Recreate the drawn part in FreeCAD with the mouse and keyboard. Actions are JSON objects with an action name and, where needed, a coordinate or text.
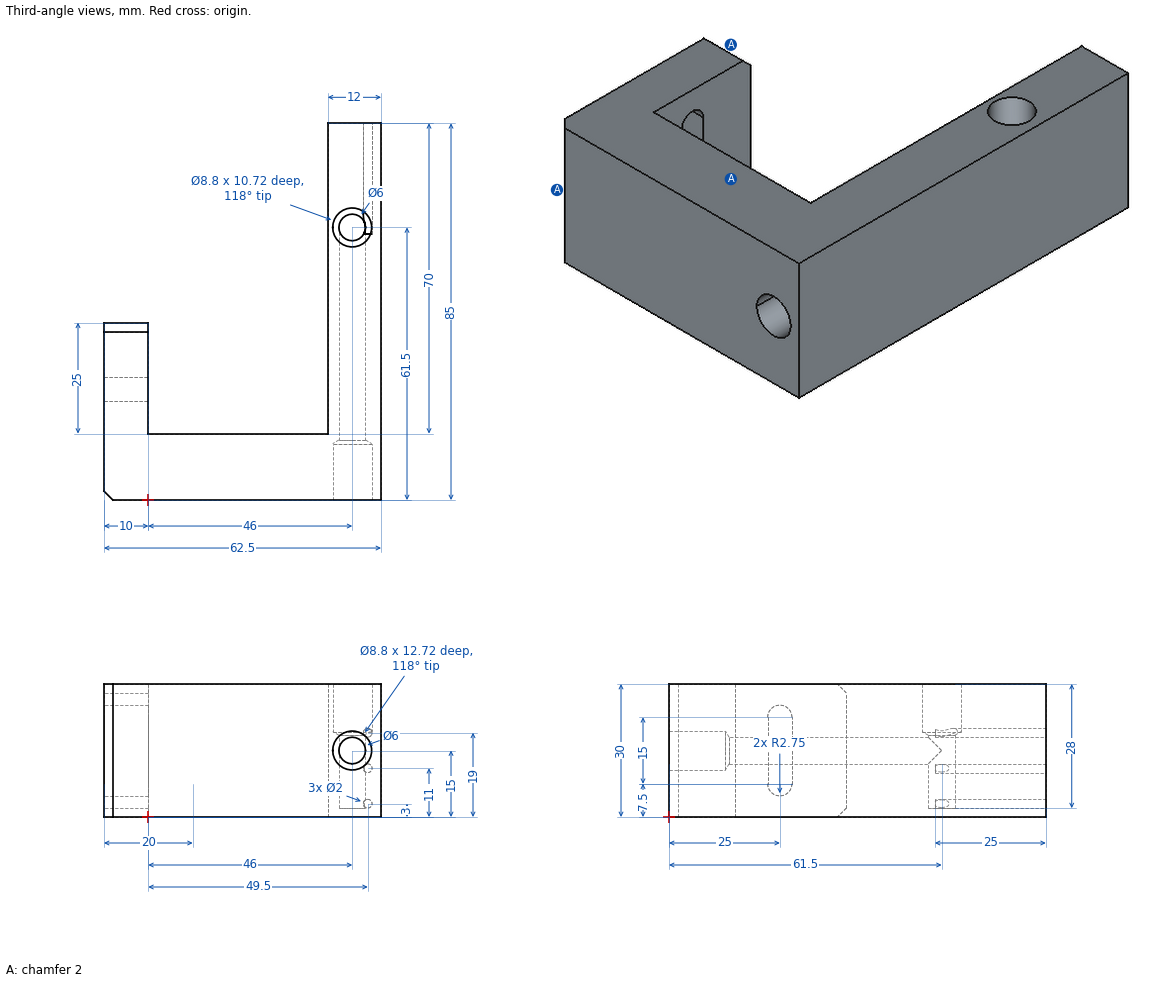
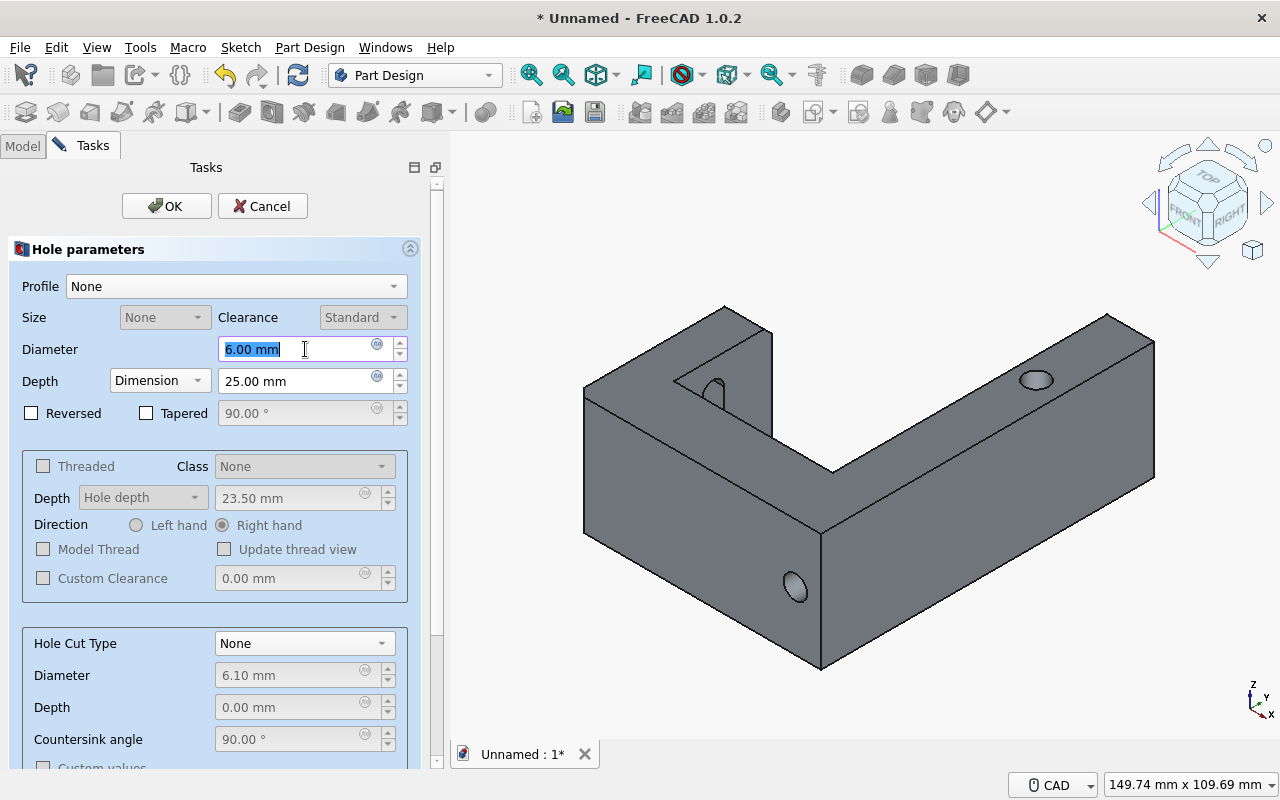
{"action": "type", "text": "8.8"}
{"action": "key", "text": "Tab"}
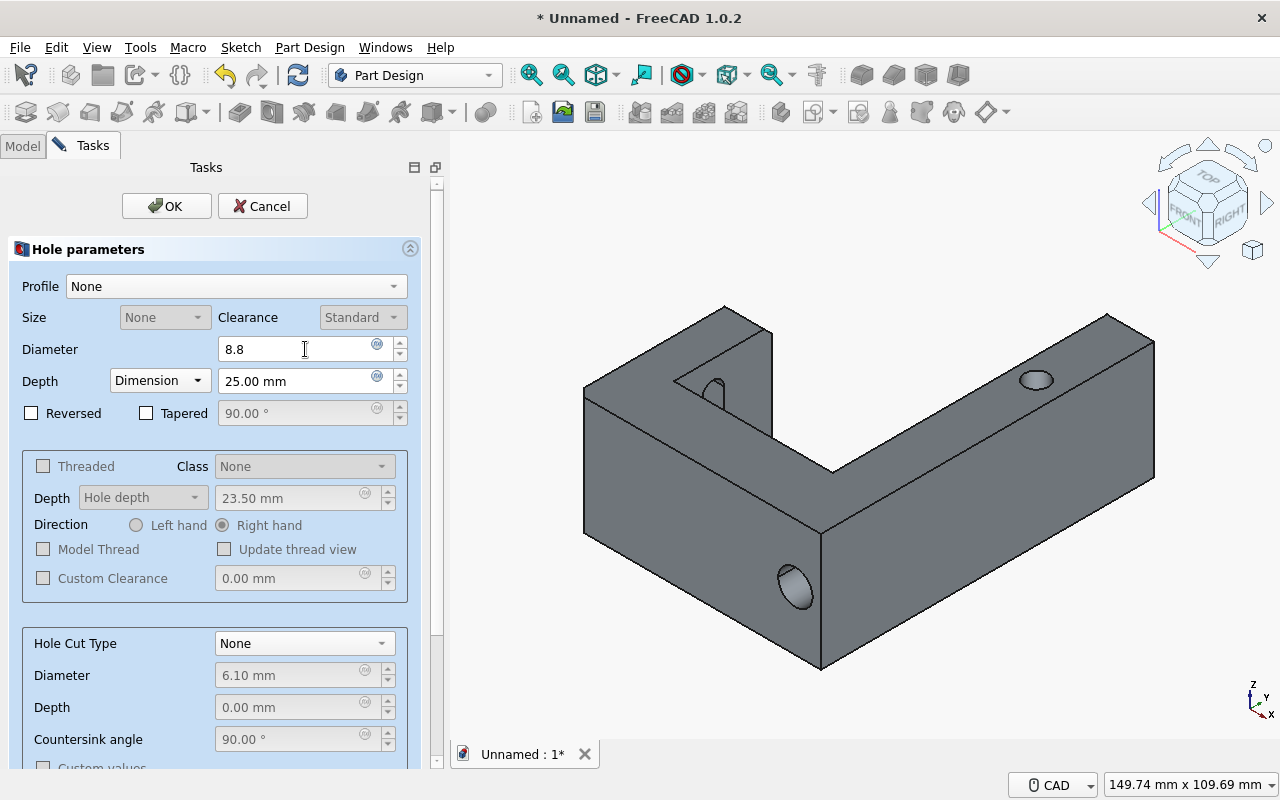
{"action": "triple_click", "coordinate": [305, 381]}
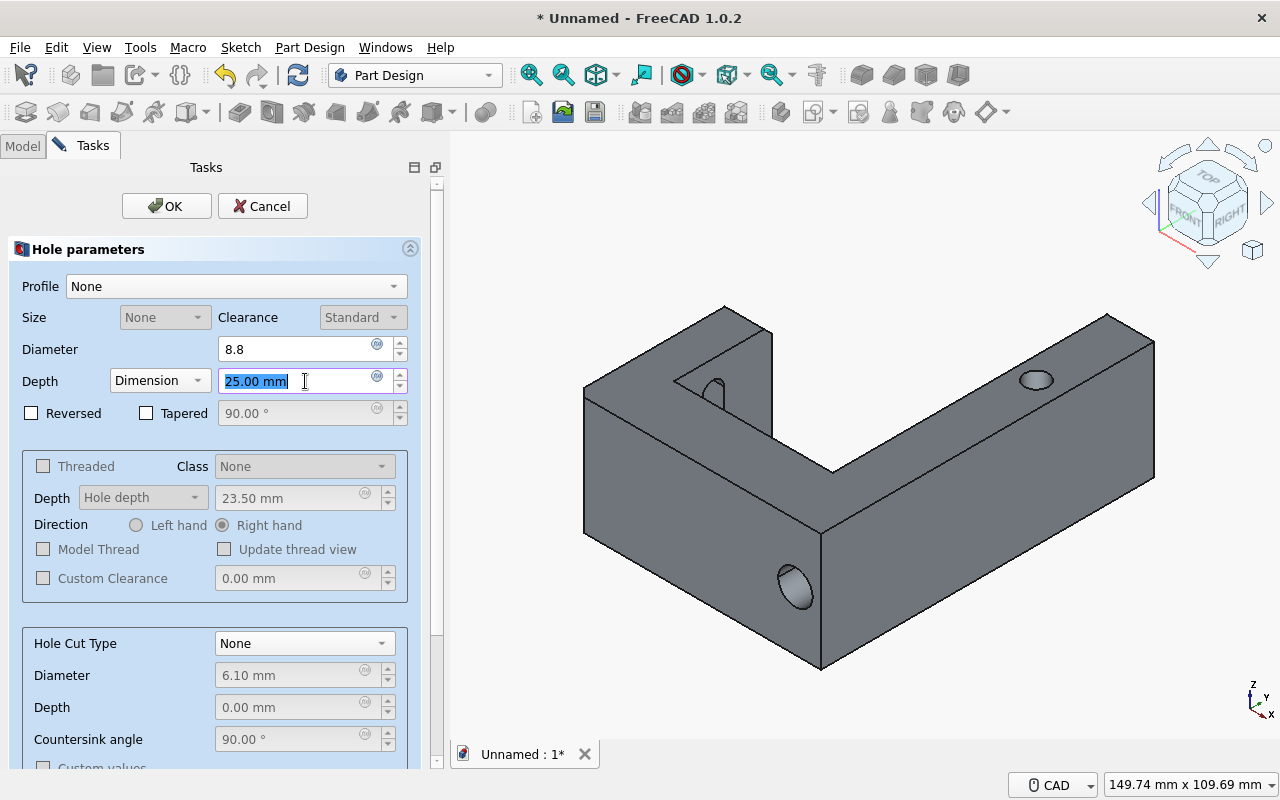
{"action": "type", "text": "12.72"}
{"action": "key", "text": "Tab"}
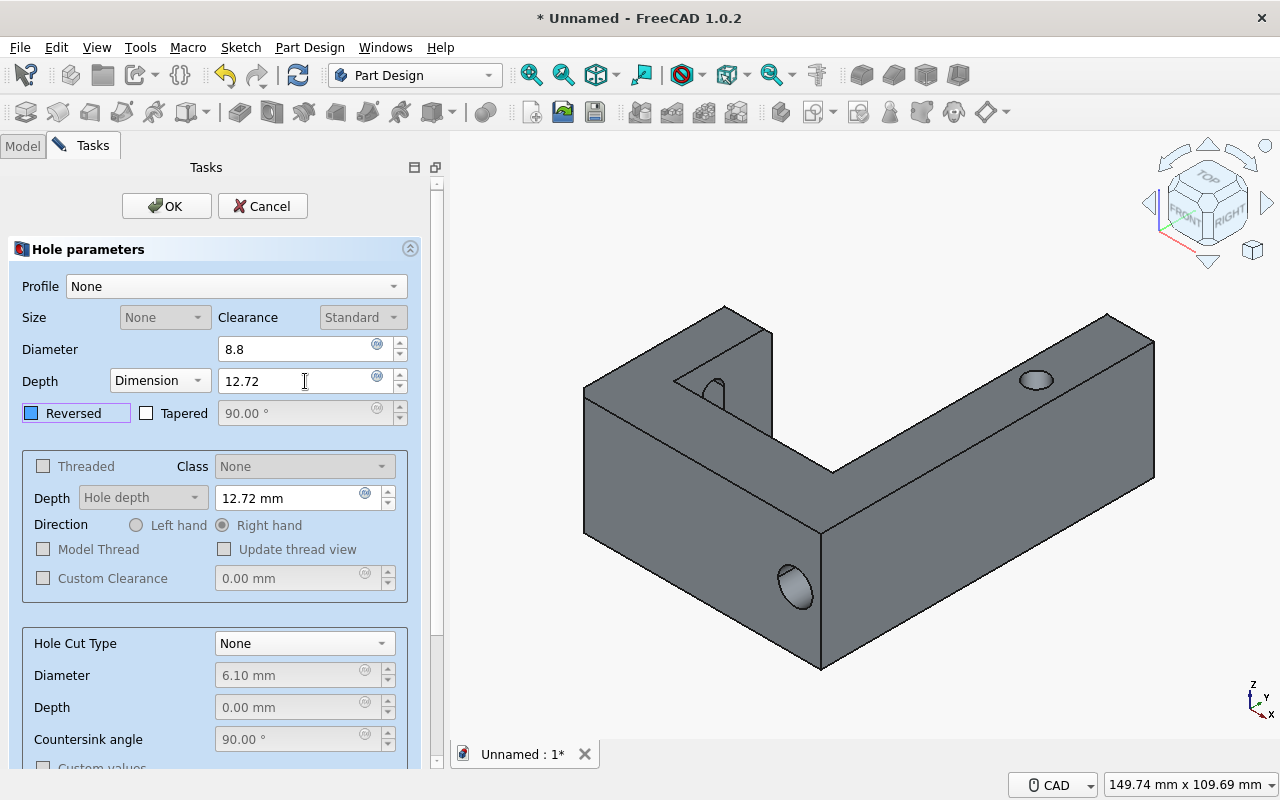
{"action": "left_click", "coordinate": [167, 206]}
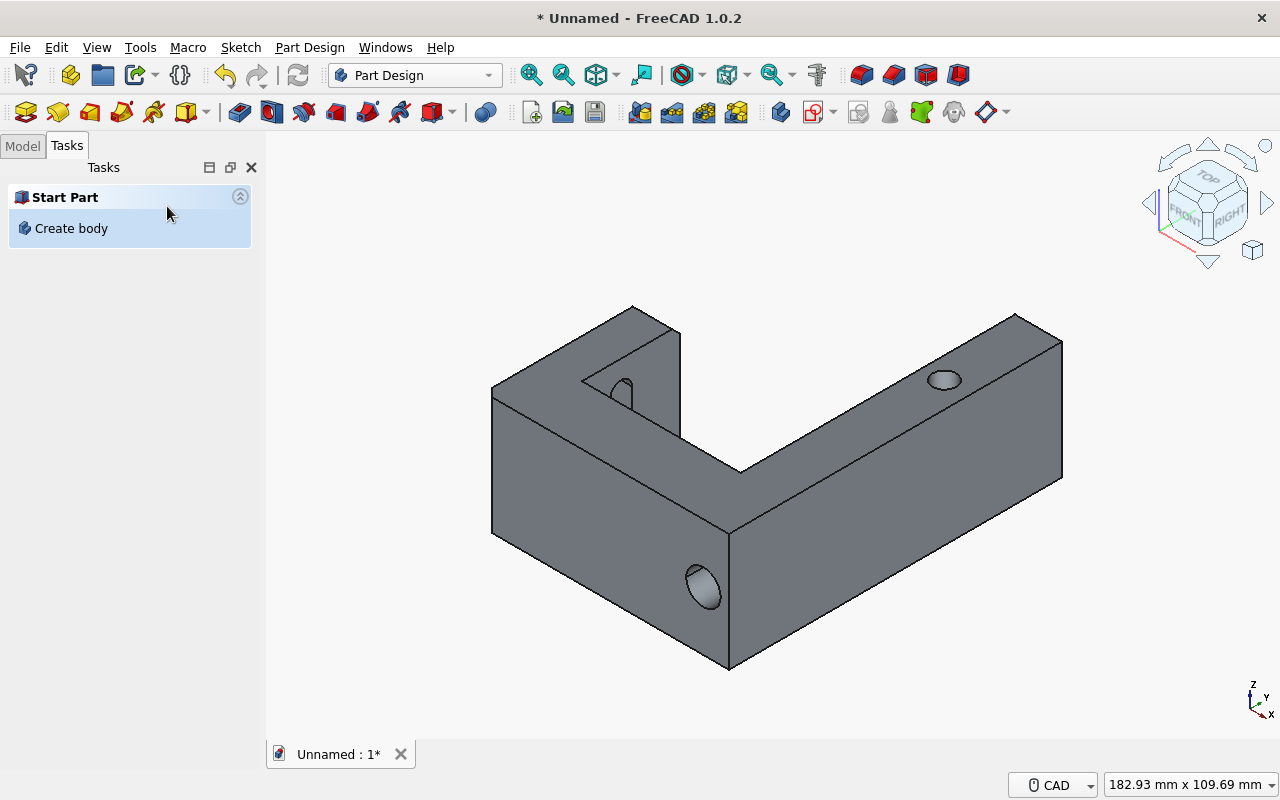
{"action": "left_click", "coordinate": [700, 489]}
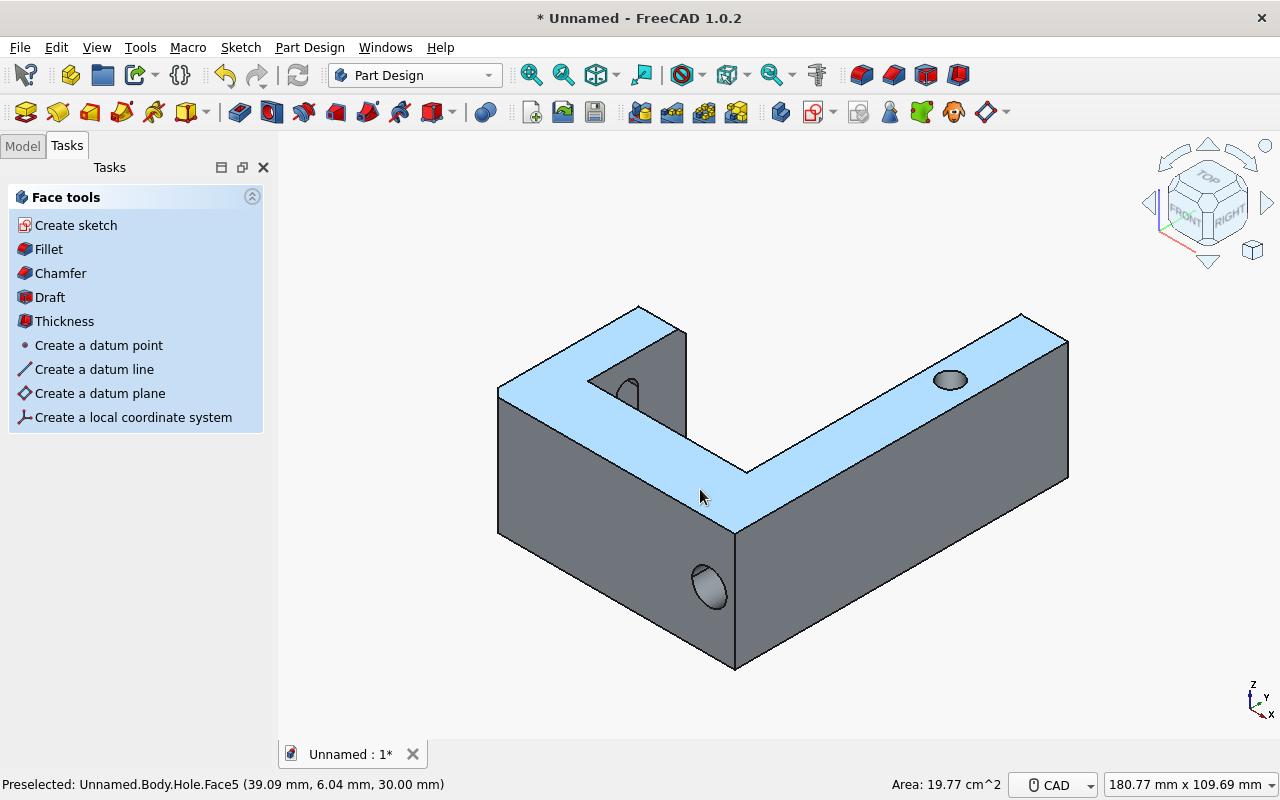
{"action": "left_click", "coordinate": [814, 112]}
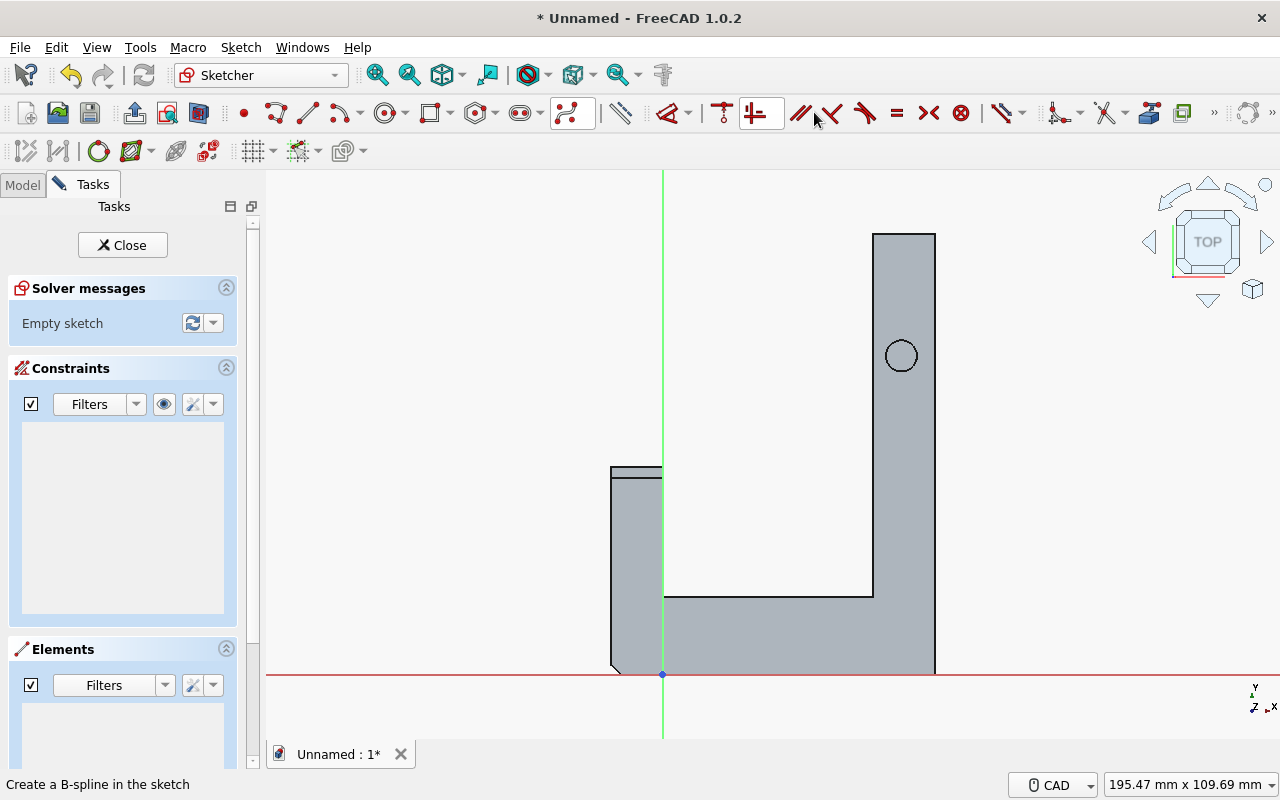
{"action": "scroll", "coordinate": [932, 341], "scroll_direction": "up", "scroll_amount": 10}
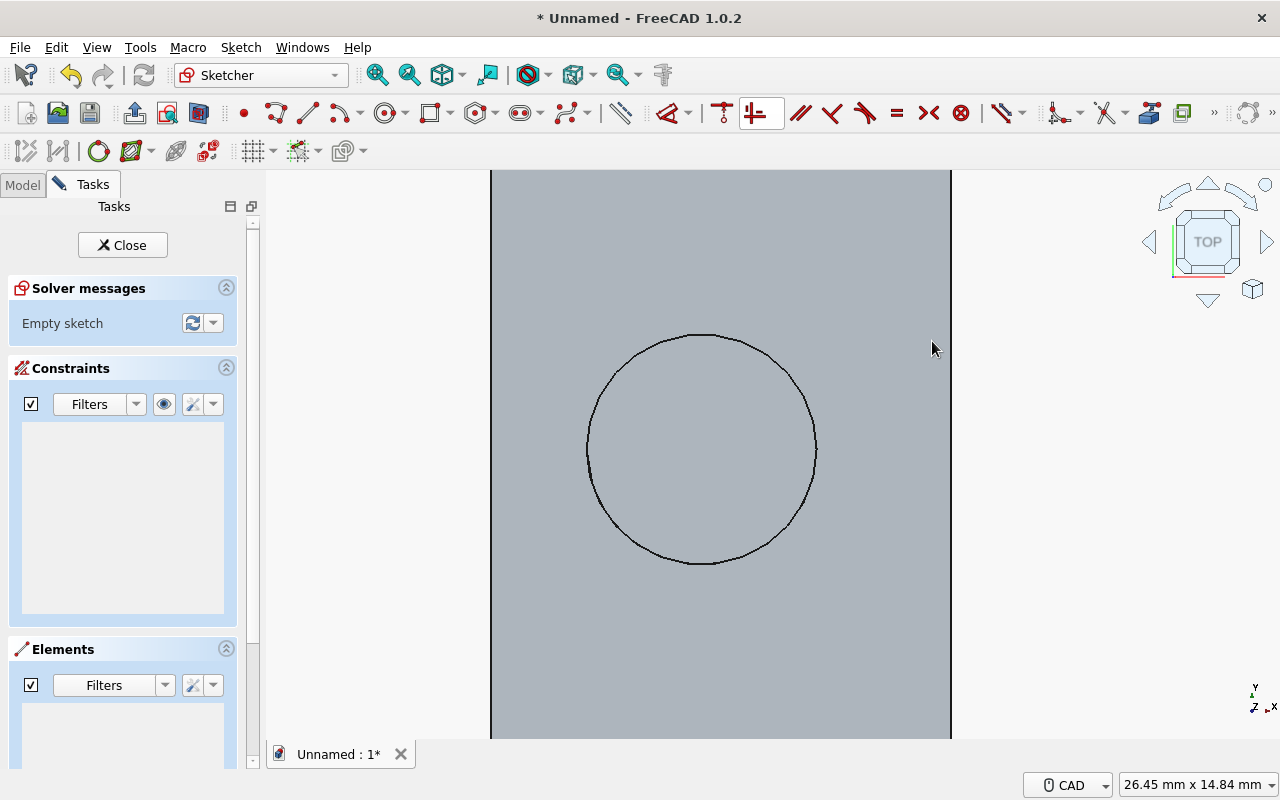
{"action": "left_click", "coordinate": [386, 114]}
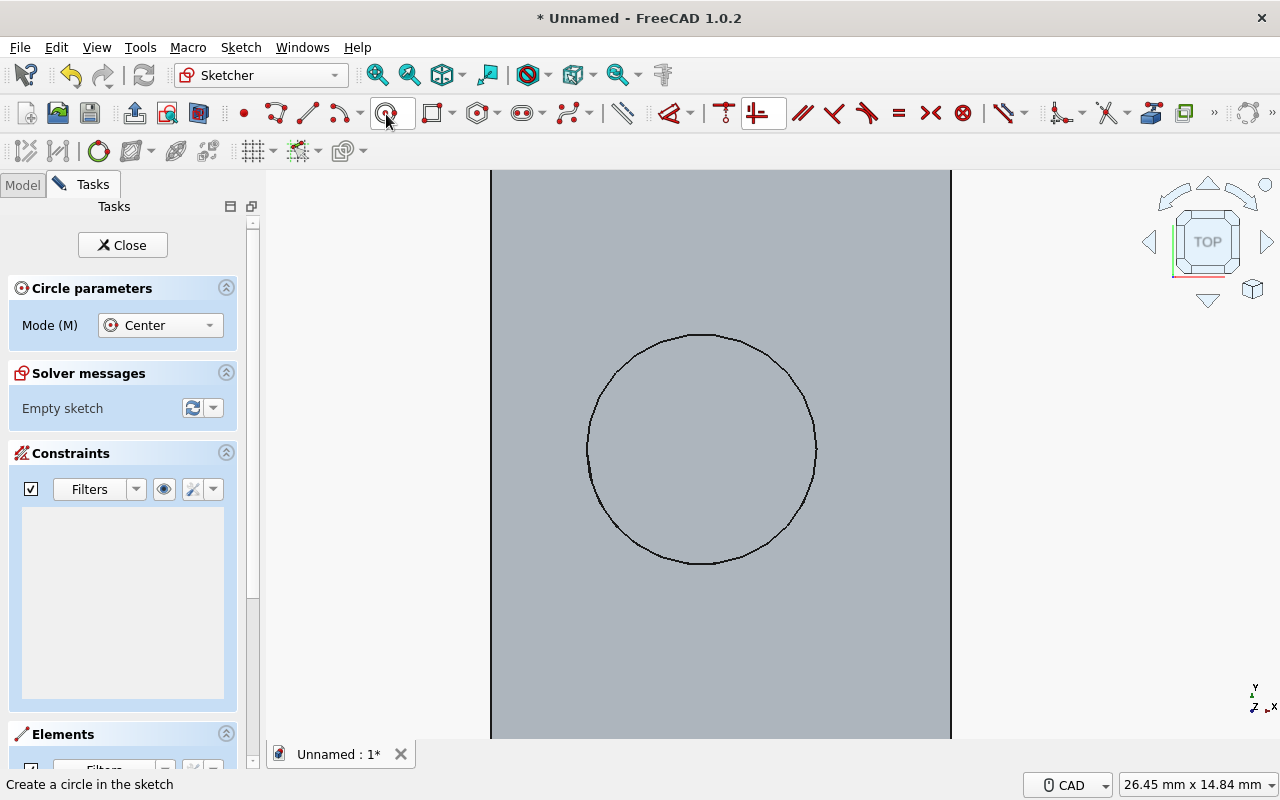
{"action": "left_click", "coordinate": [702, 449]}
{"action": "mouse_move", "coordinate": [821, 330]}